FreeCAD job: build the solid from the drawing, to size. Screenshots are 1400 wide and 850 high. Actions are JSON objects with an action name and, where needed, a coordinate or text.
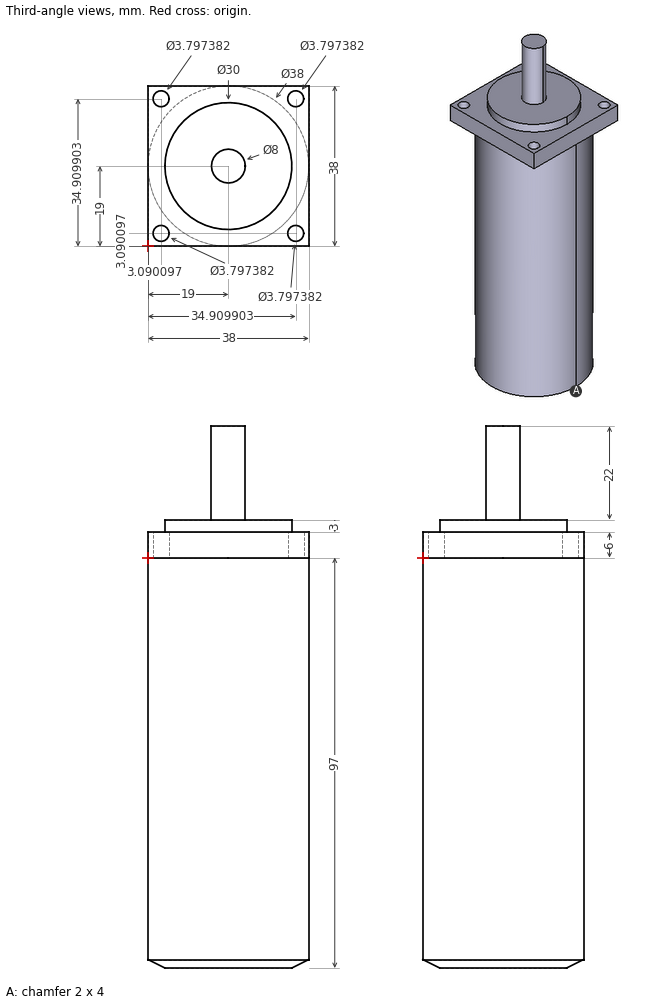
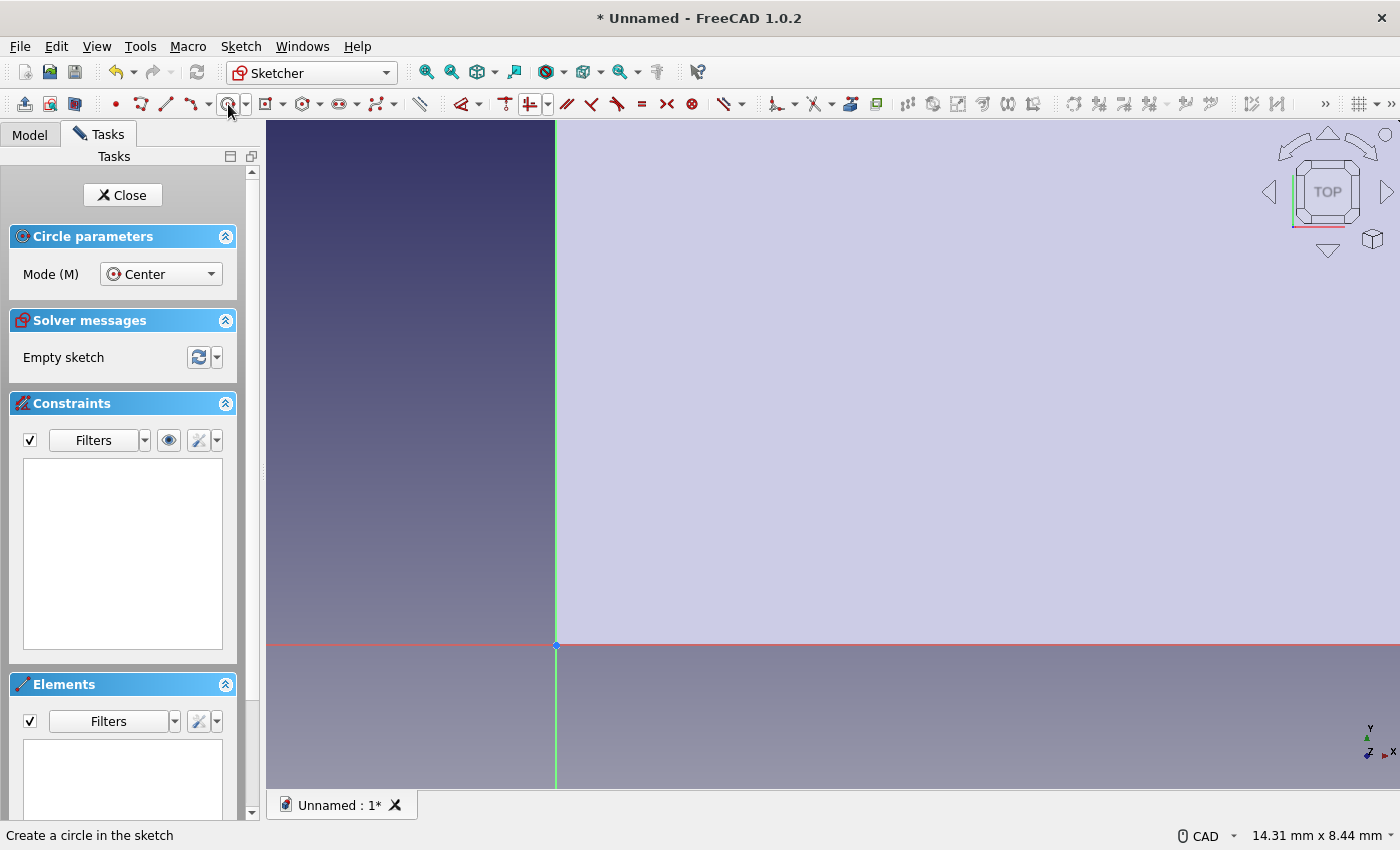
{"action": "left_click", "coordinate": [801, 401]}
{"action": "mouse_move", "coordinate": [908, 294]}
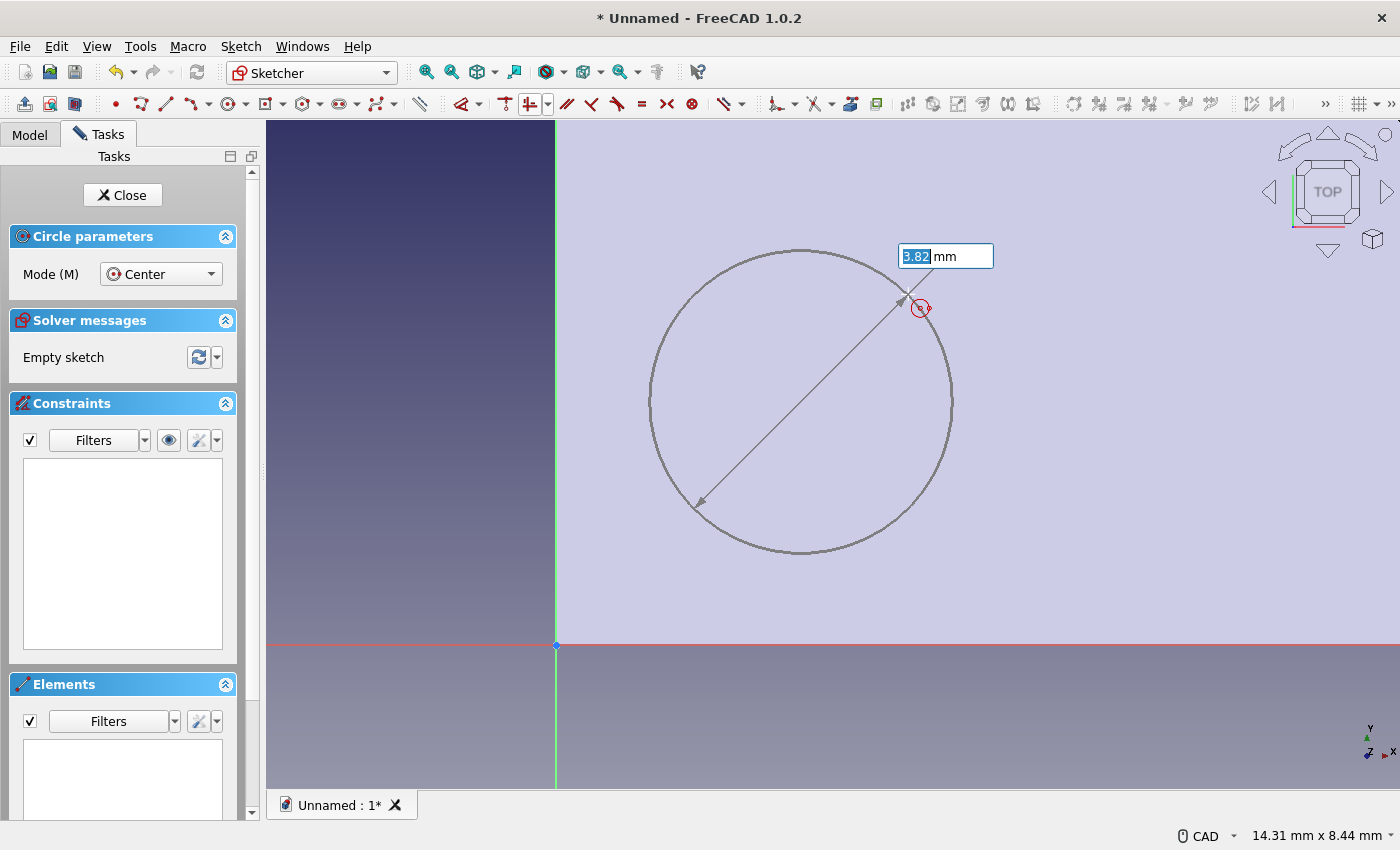
{"action": "type", "text": "3.797382"}
{"action": "key", "text": "Return"}
{"action": "key", "text": "Escape"}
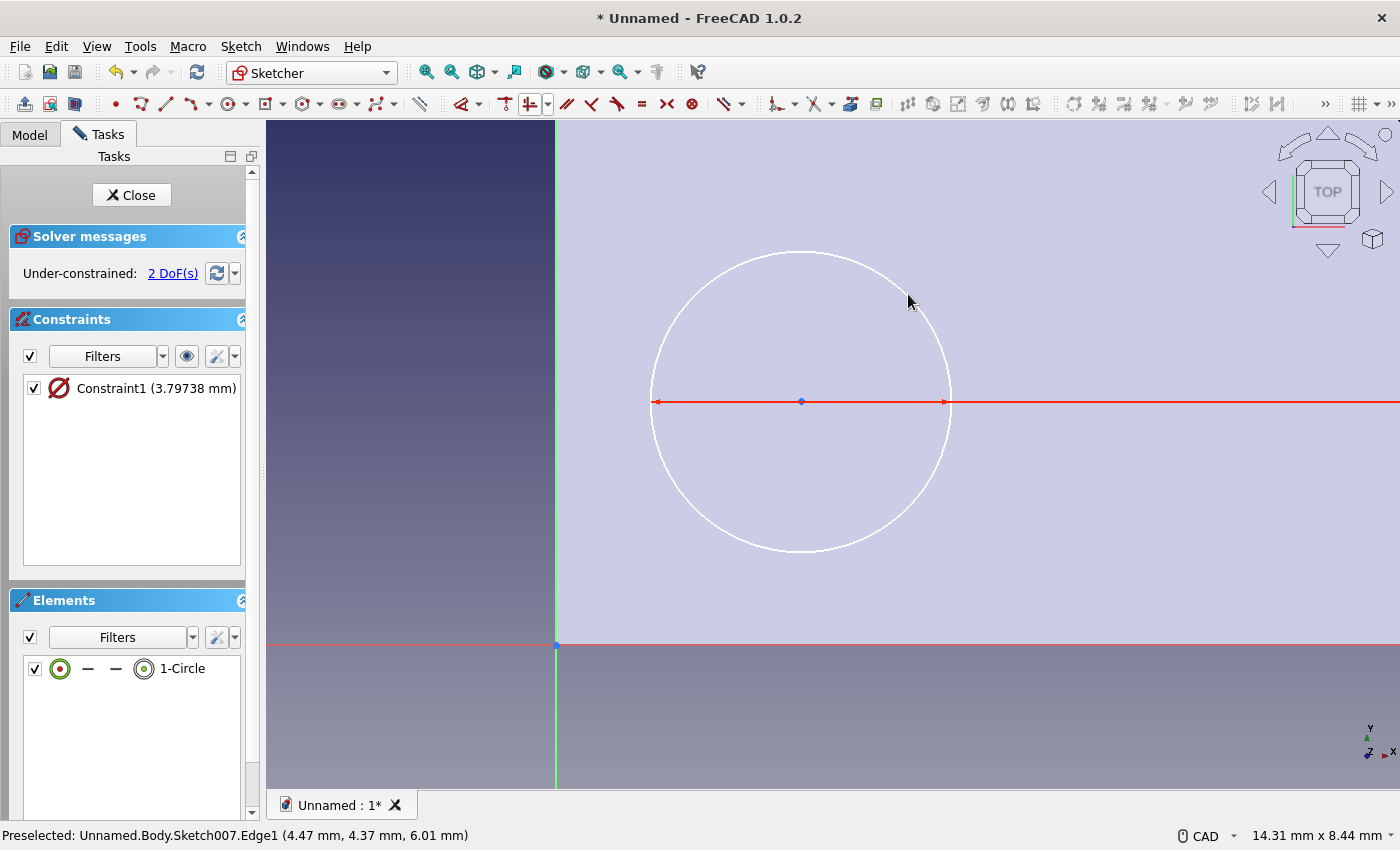
{"action": "left_click", "coordinate": [460, 104]}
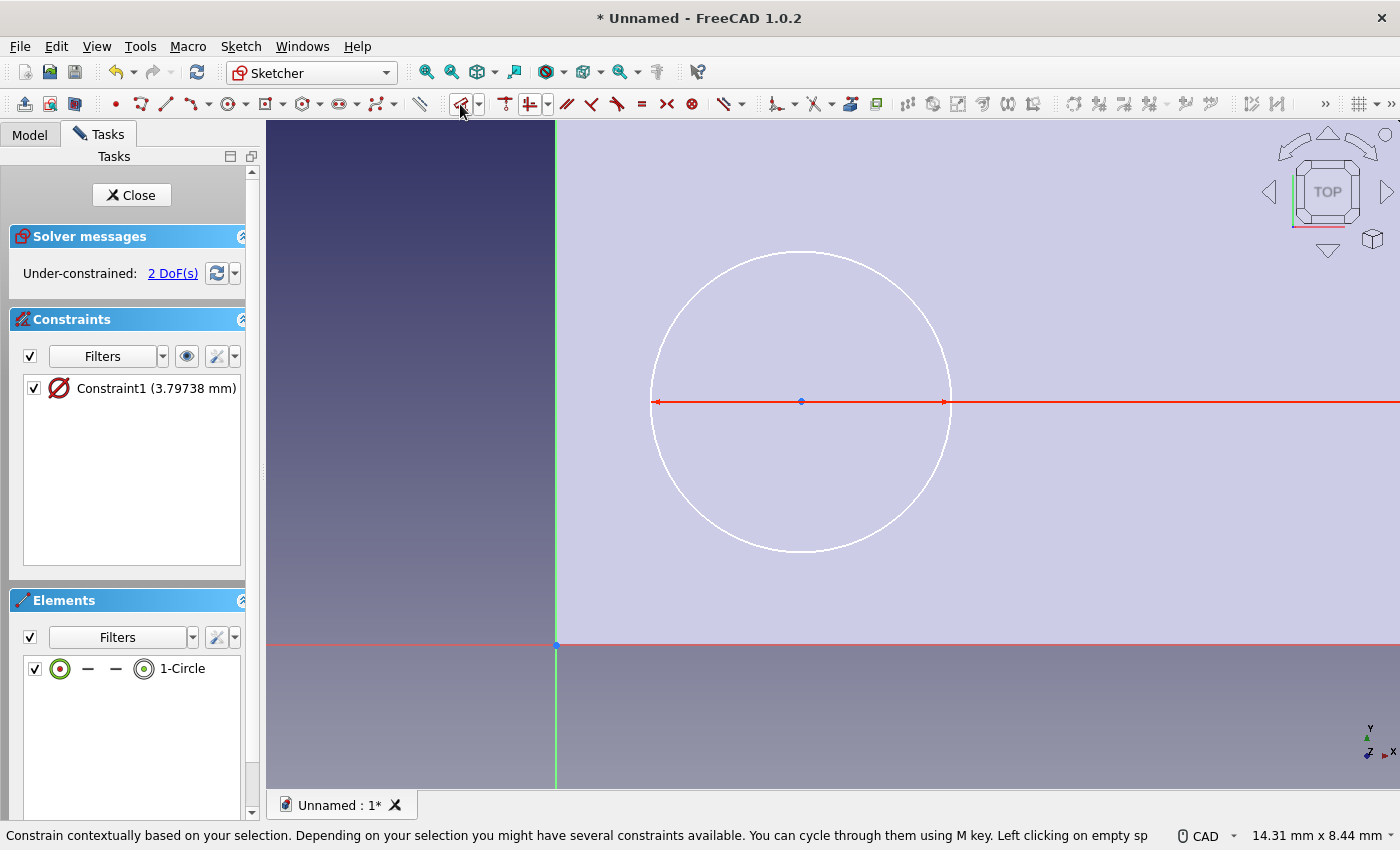
{"action": "left_click", "coordinate": [801, 402]}
{"action": "left_click", "coordinate": [679, 679]}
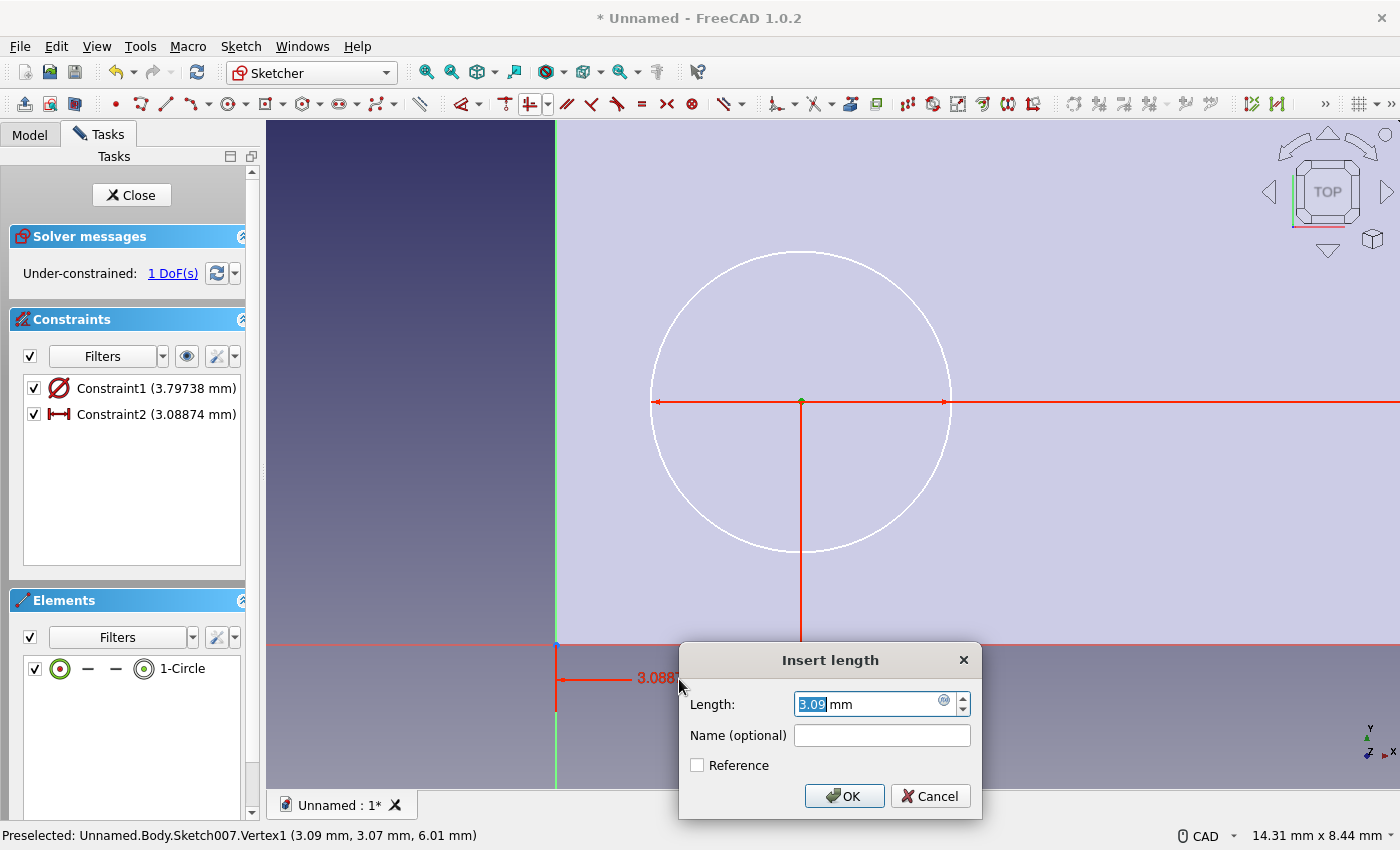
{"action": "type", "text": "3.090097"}
{"action": "key", "text": "Return"}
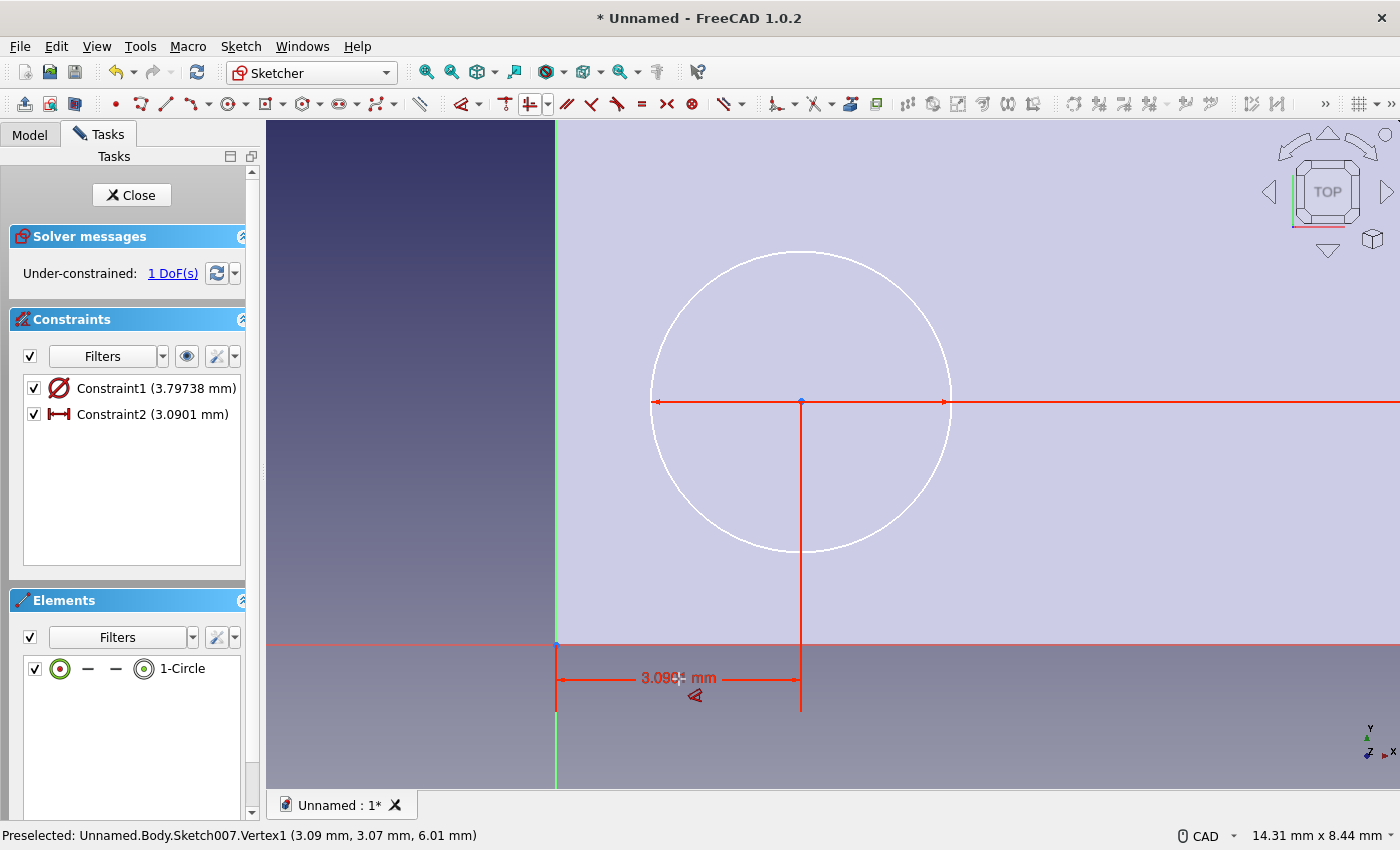
{"action": "left_click", "coordinate": [801, 402]}
{"action": "left_click", "coordinate": [522, 524]}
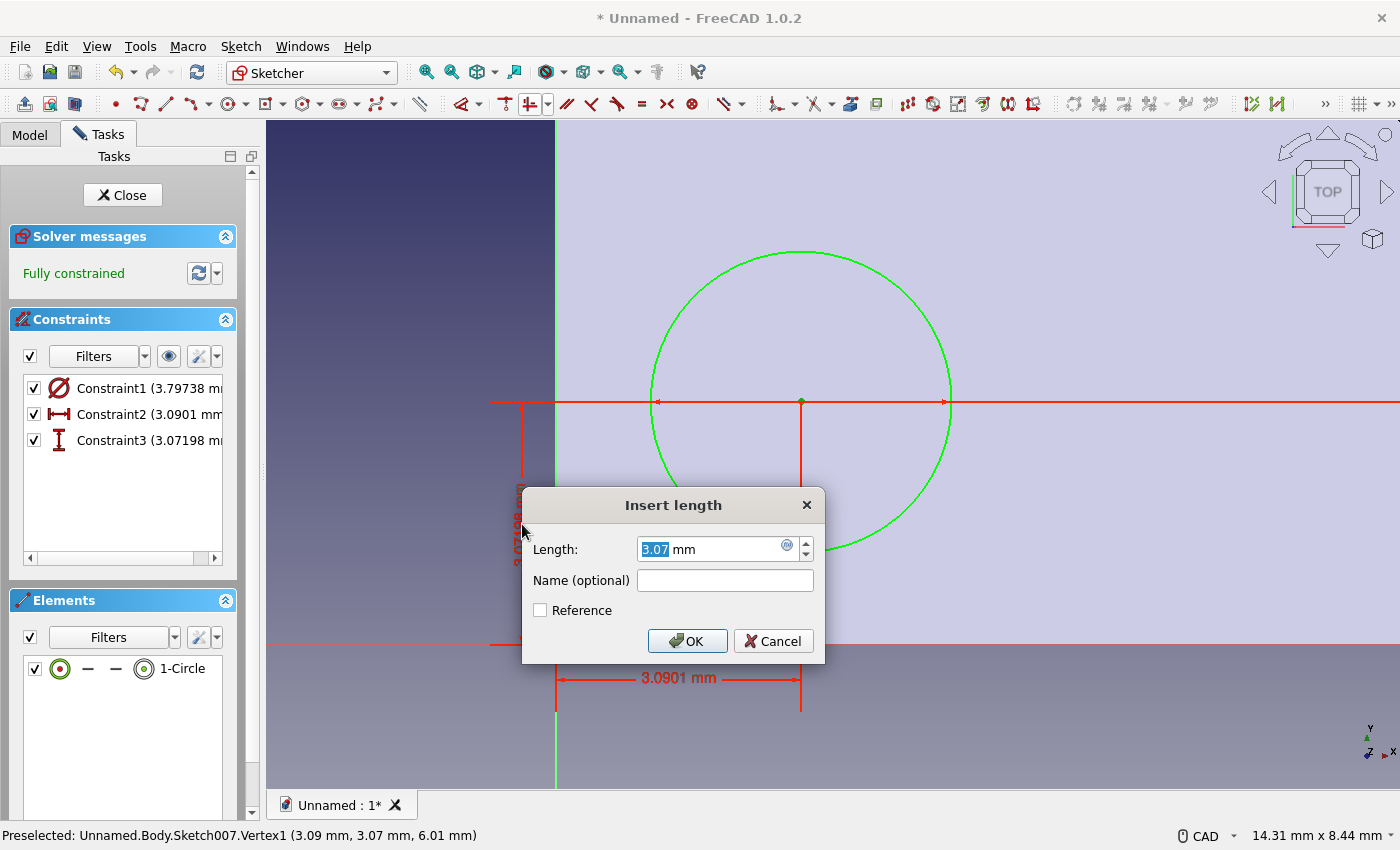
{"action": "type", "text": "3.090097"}
{"action": "key", "text": "Return"}
{"action": "key", "text": "Escape"}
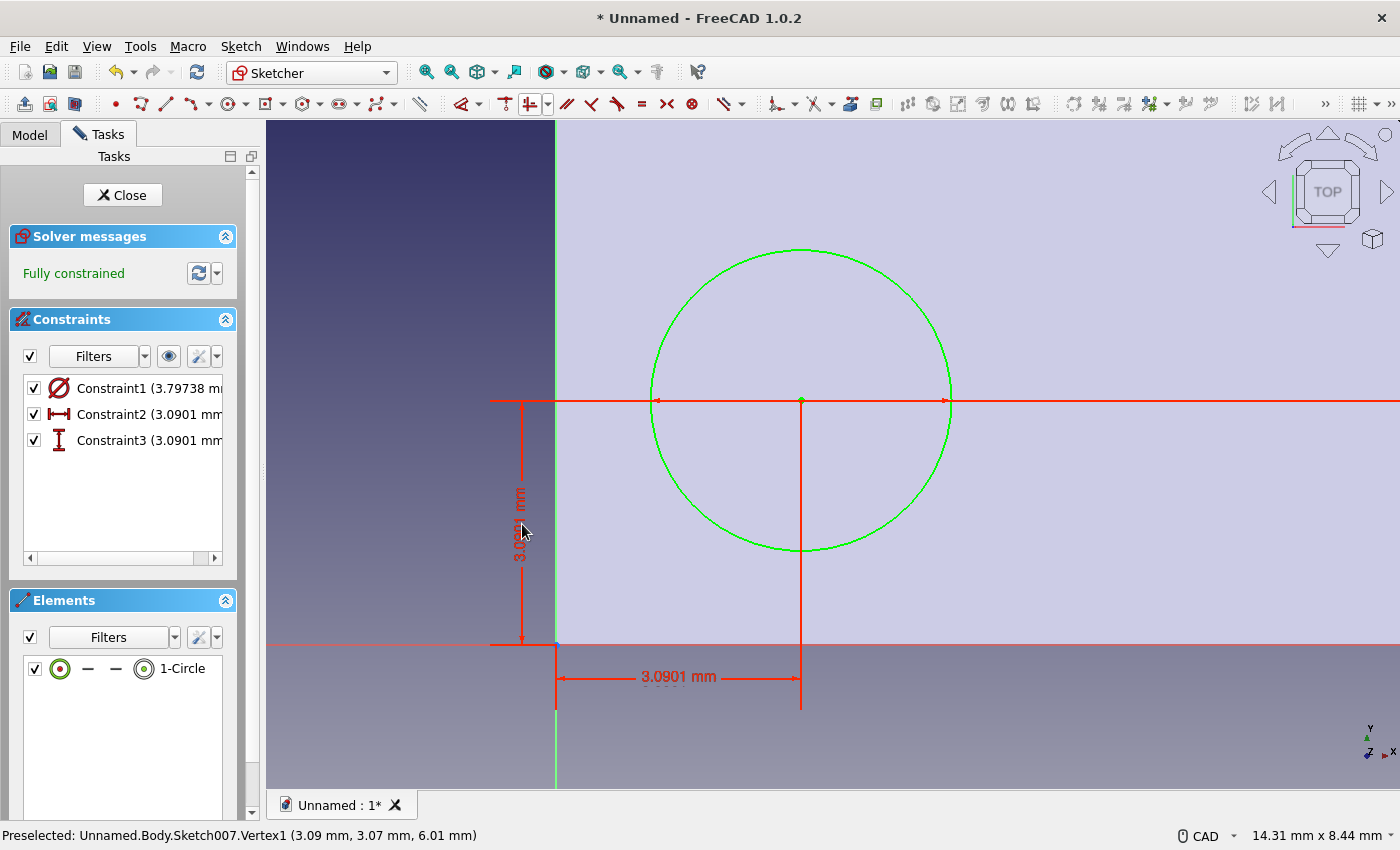
{"action": "left_click", "coordinate": [123, 195]}